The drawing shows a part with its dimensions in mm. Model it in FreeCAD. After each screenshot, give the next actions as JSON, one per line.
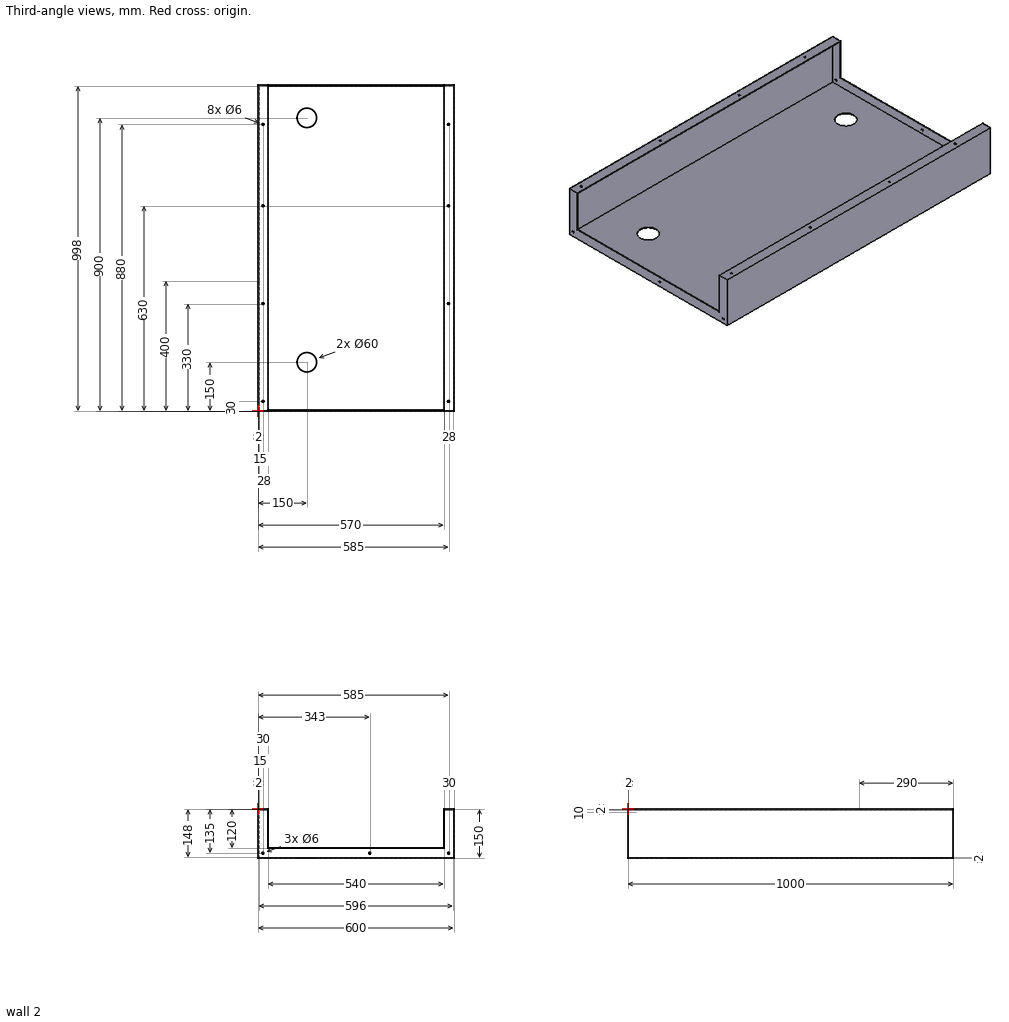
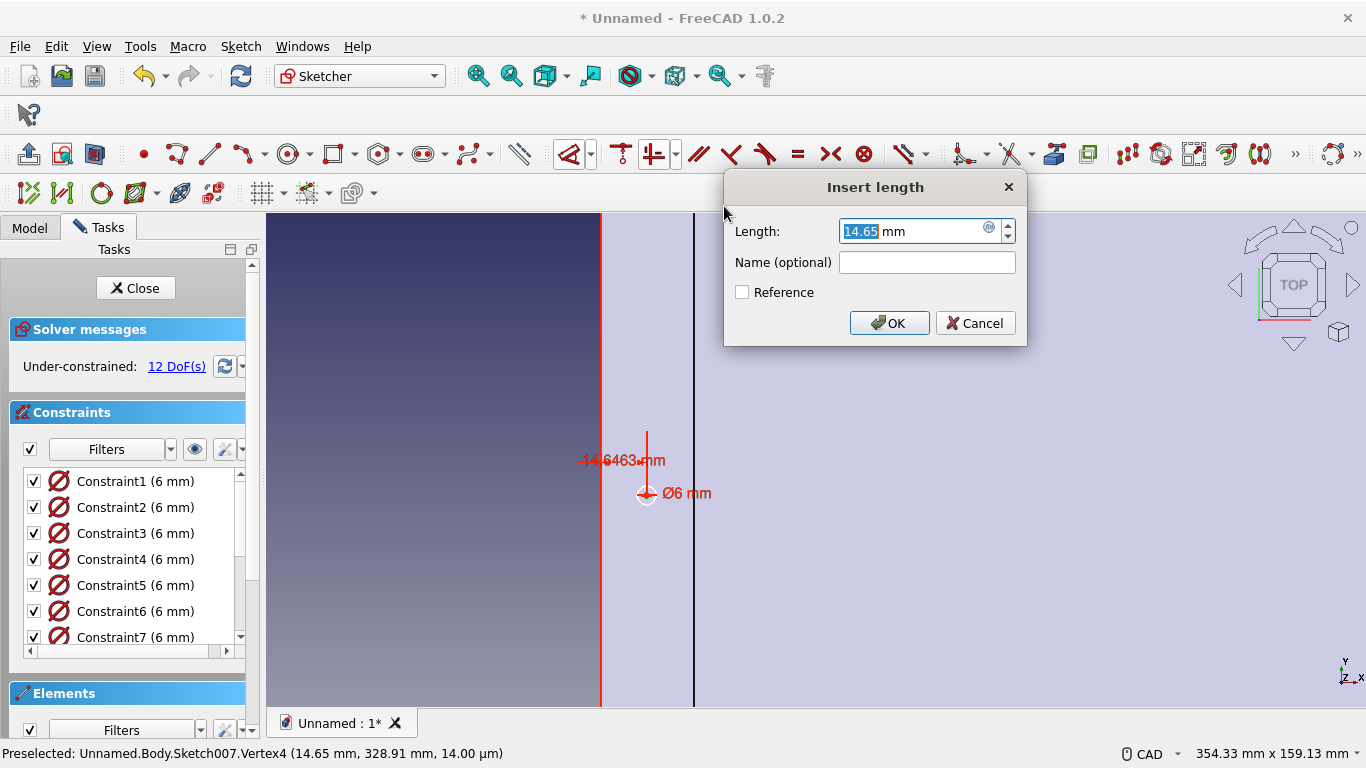
{"action": "type", "text": "15"}
{"action": "key", "text": "Return"}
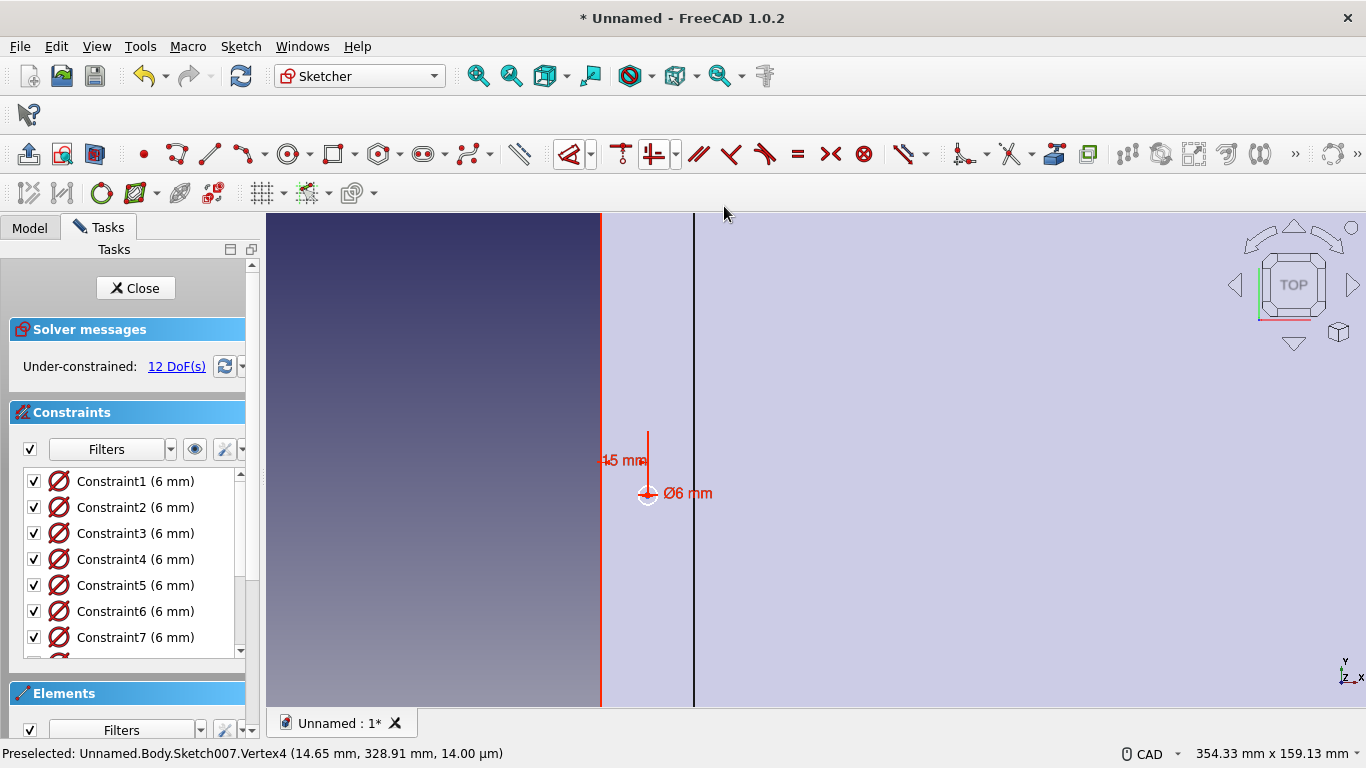
{"action": "scroll", "coordinate": [652, 499], "scroll_direction": "down", "scroll_amount": 11}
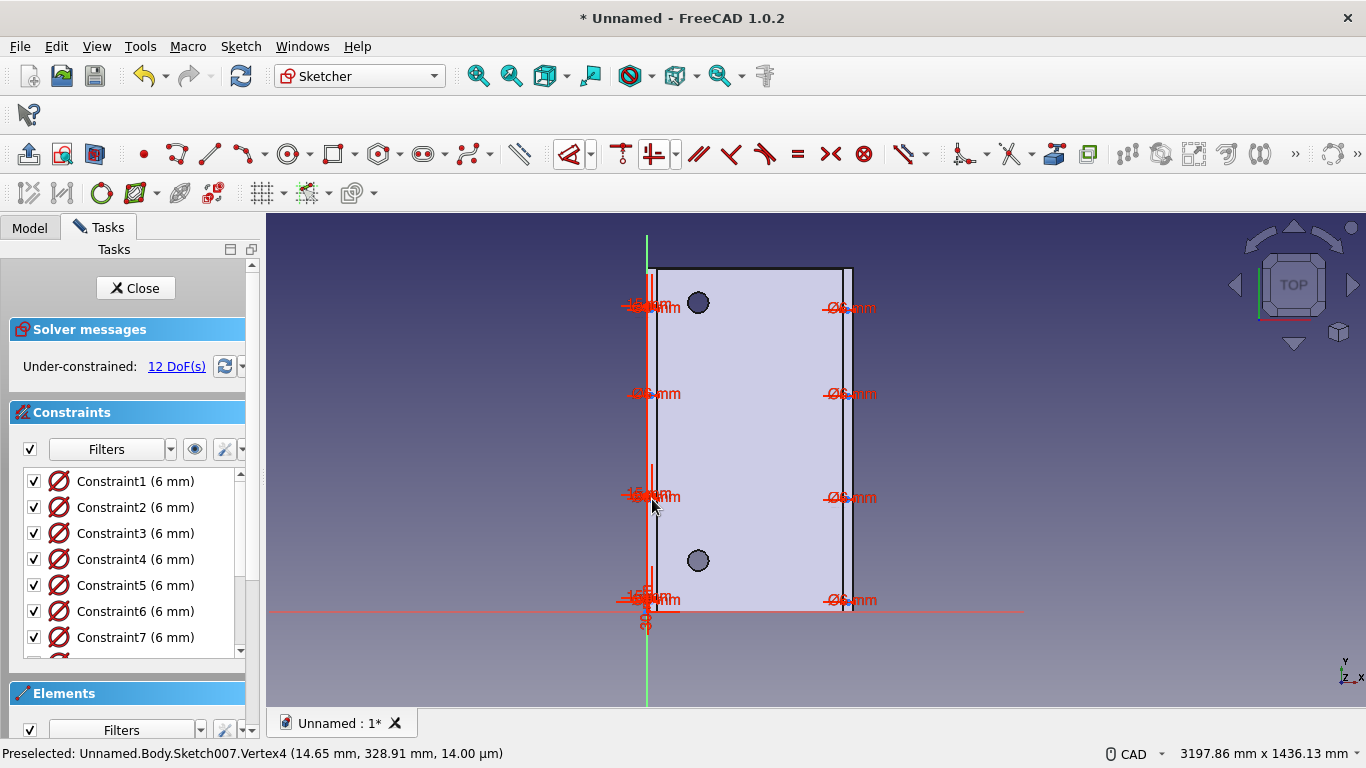
{"action": "scroll", "coordinate": [652, 396], "scroll_direction": "up", "scroll_amount": 11}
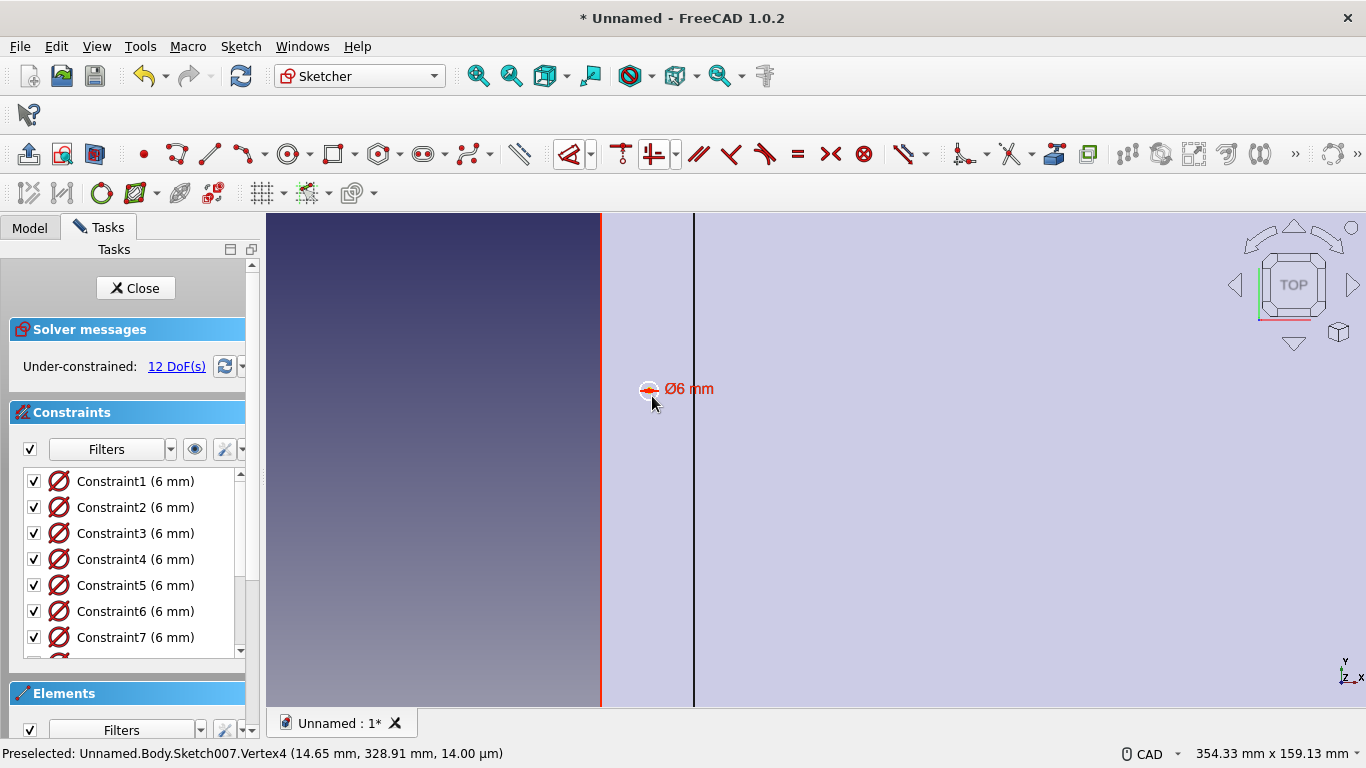
{"action": "left_click", "coordinate": [649, 391]}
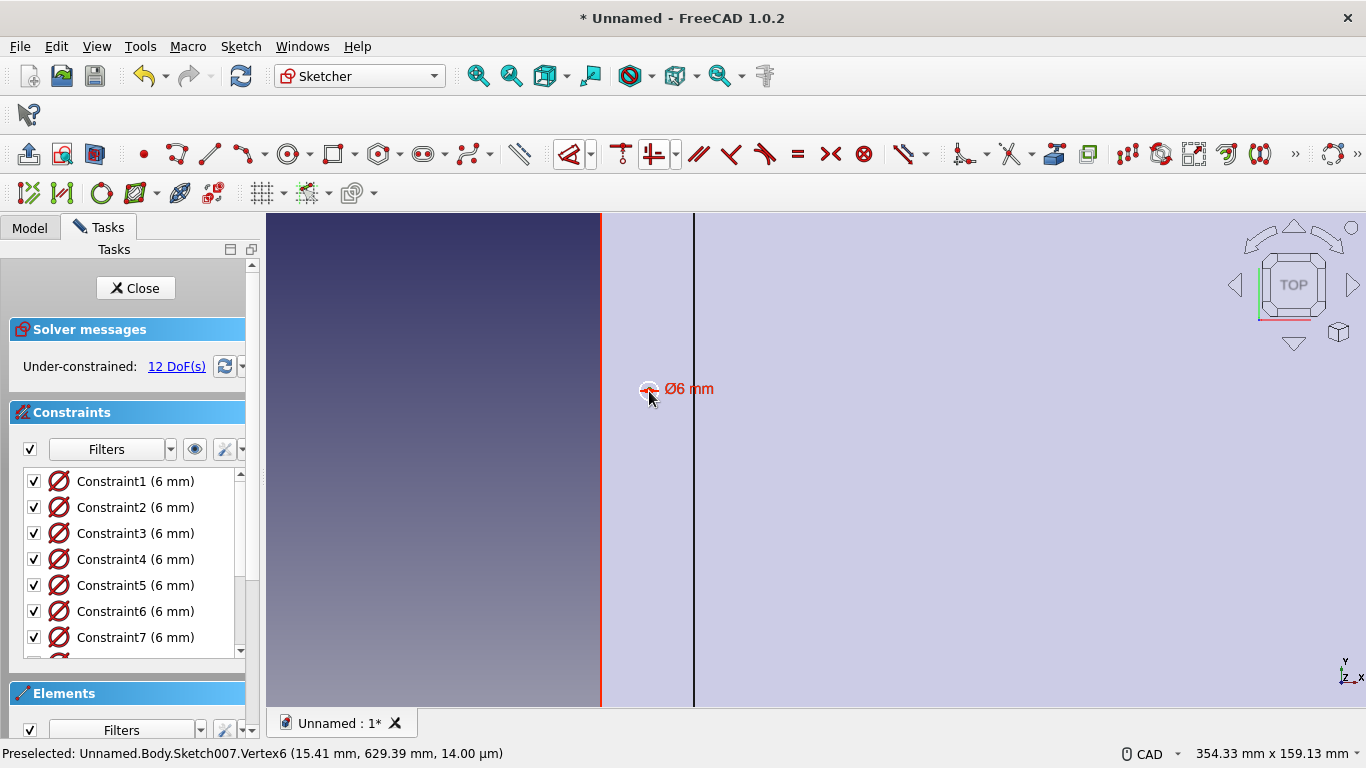
{"action": "left_click", "coordinate": [590, 154]}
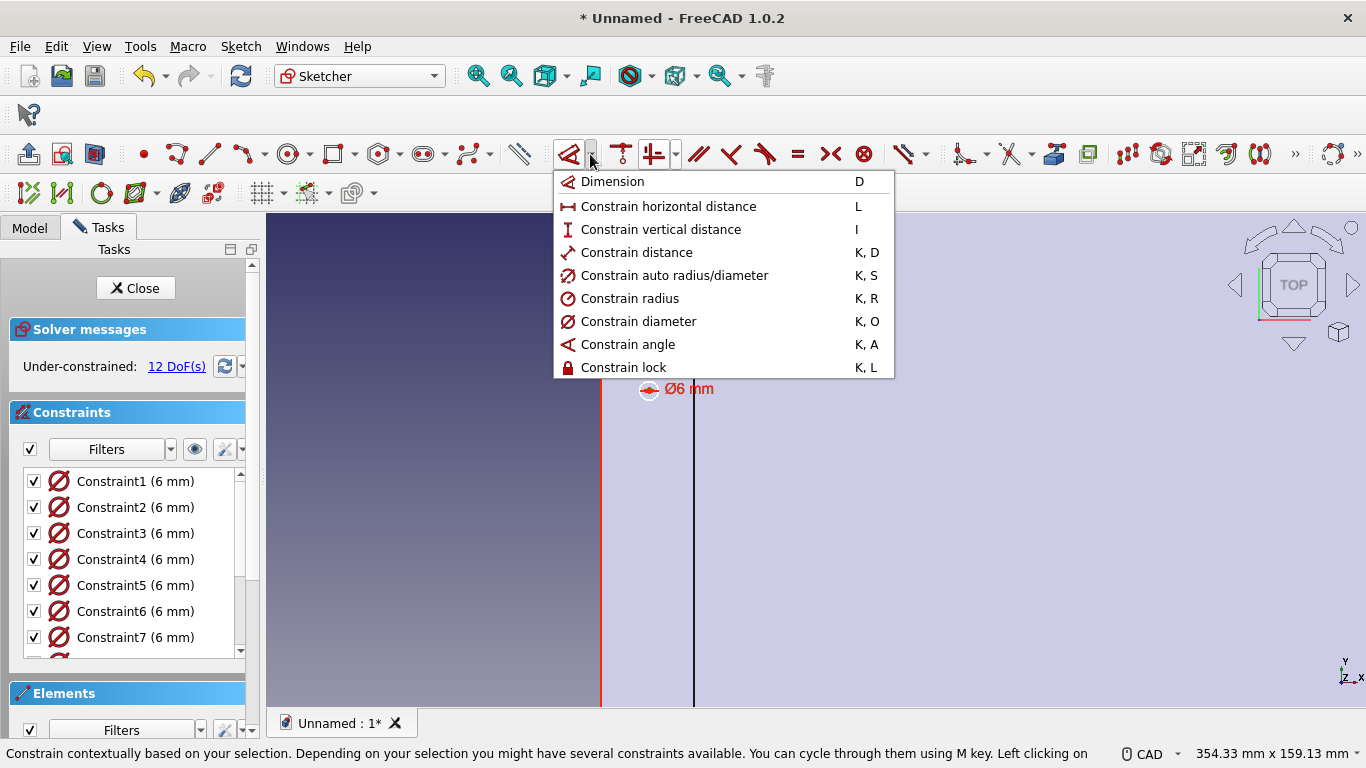
{"action": "left_click", "coordinate": [724, 206]}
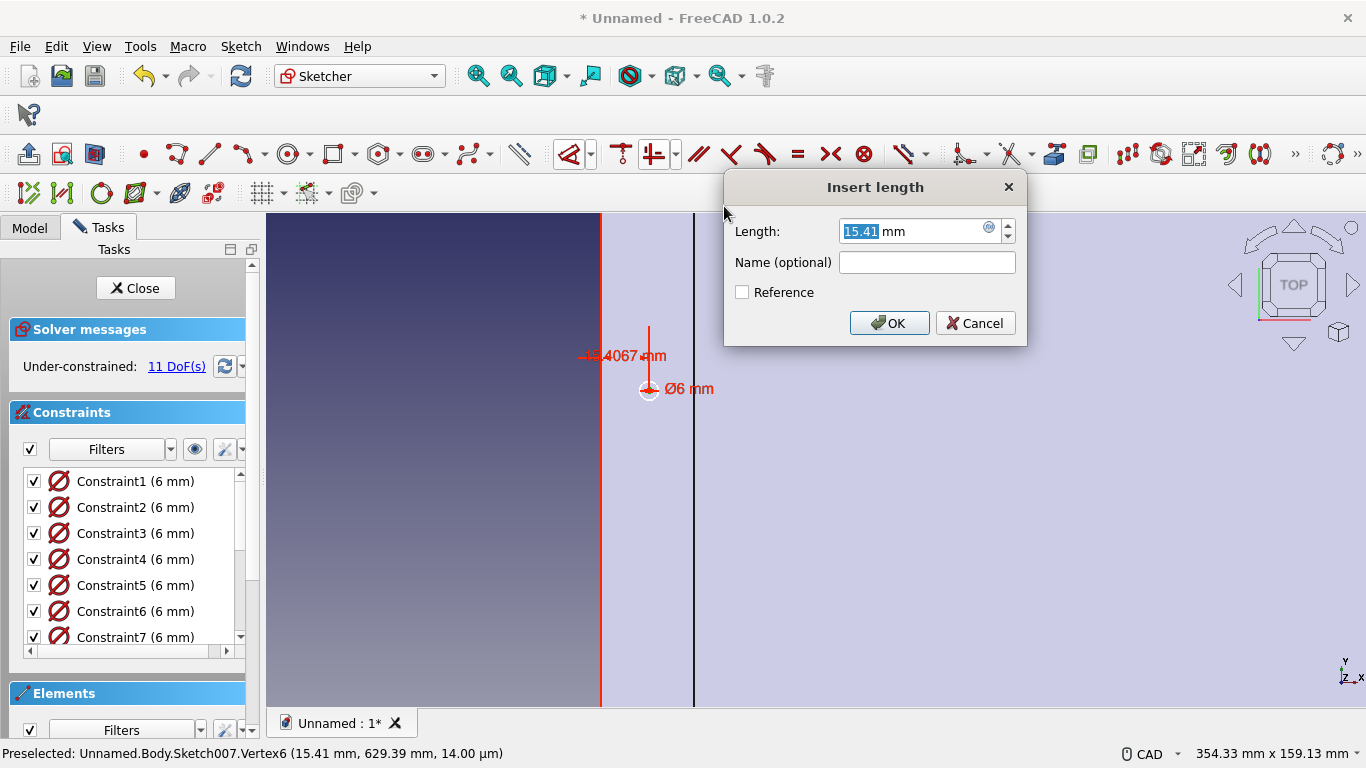
{"action": "type", "text": "15"}
{"action": "key", "text": "Return"}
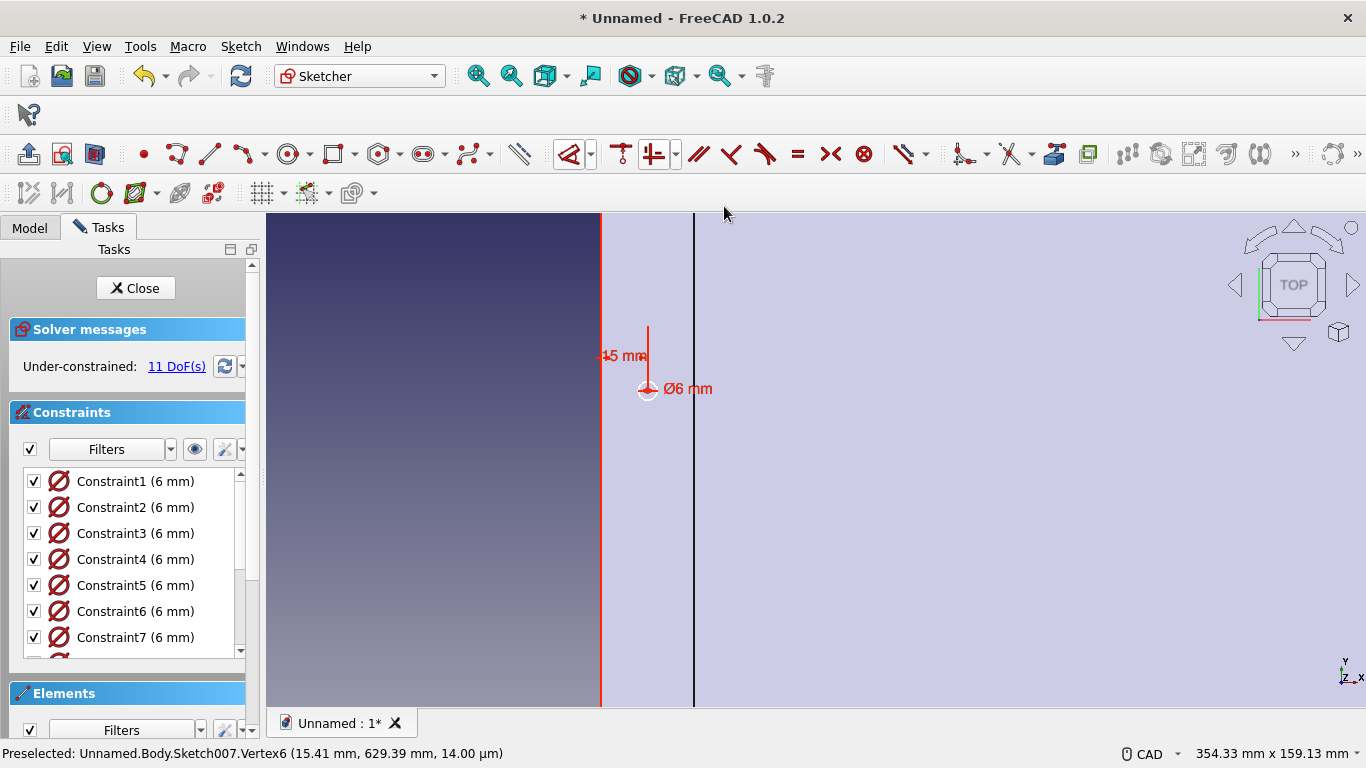
{"action": "scroll", "coordinate": [652, 396], "scroll_direction": "down", "scroll_amount": 11}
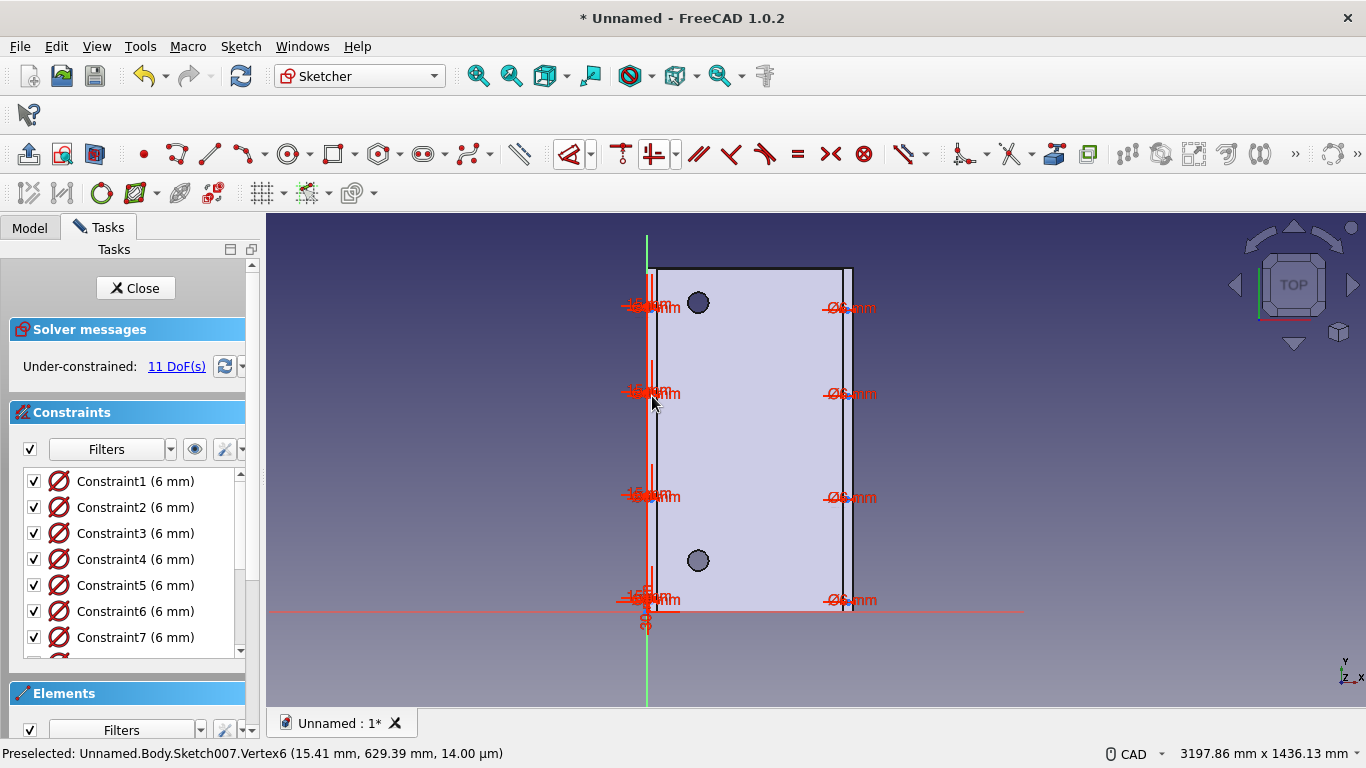
{"action": "scroll", "coordinate": [848, 602], "scroll_direction": "up", "scroll_amount": 7}